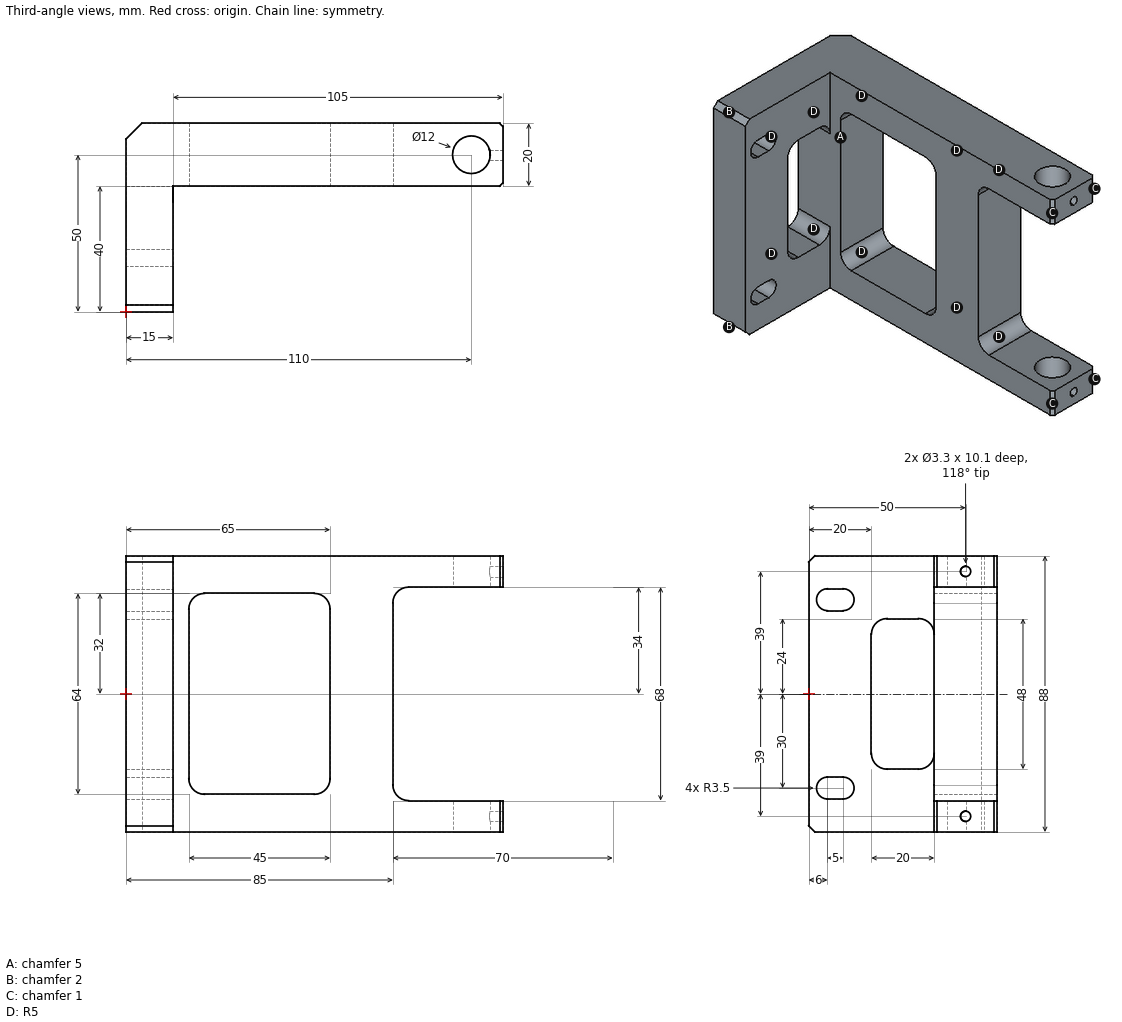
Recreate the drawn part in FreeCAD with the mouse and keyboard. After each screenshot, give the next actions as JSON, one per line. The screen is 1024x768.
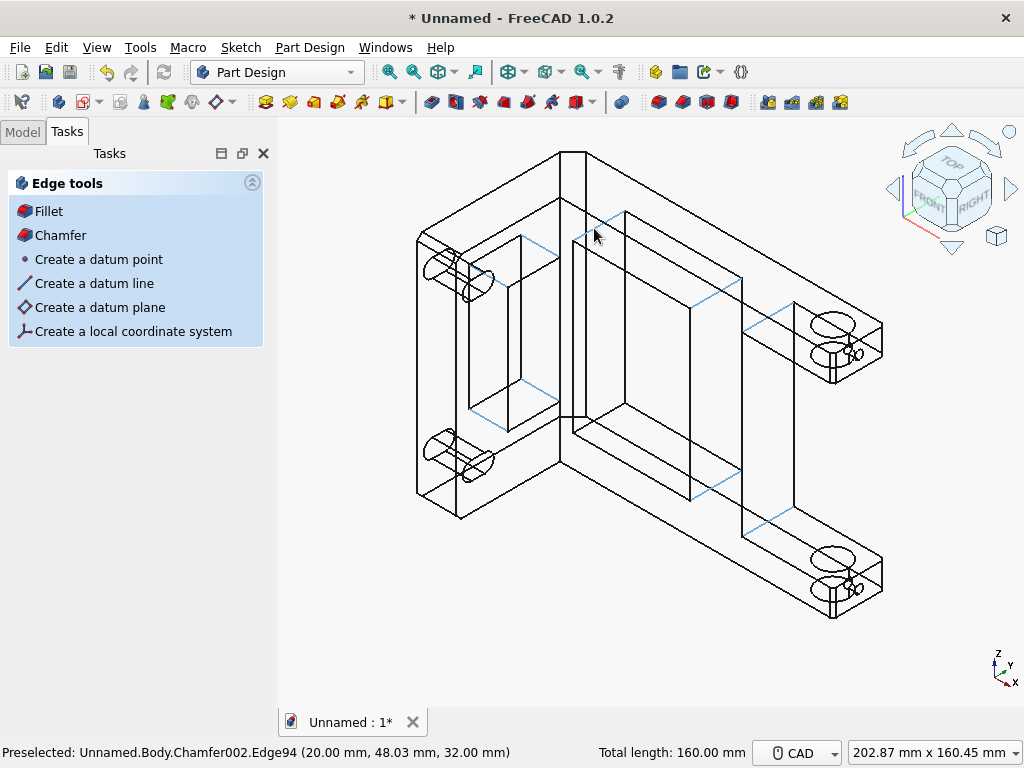
{"action": "left_click", "coordinate": [599, 417], "text": "ctrl"}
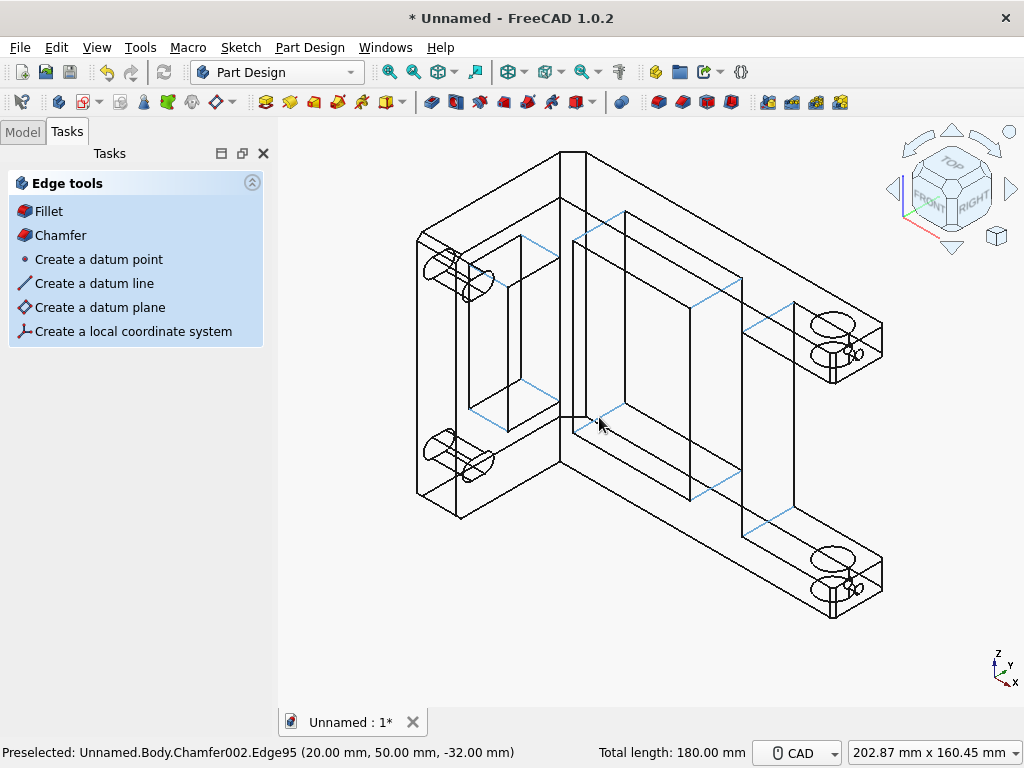
{"action": "key", "text": "v 1"}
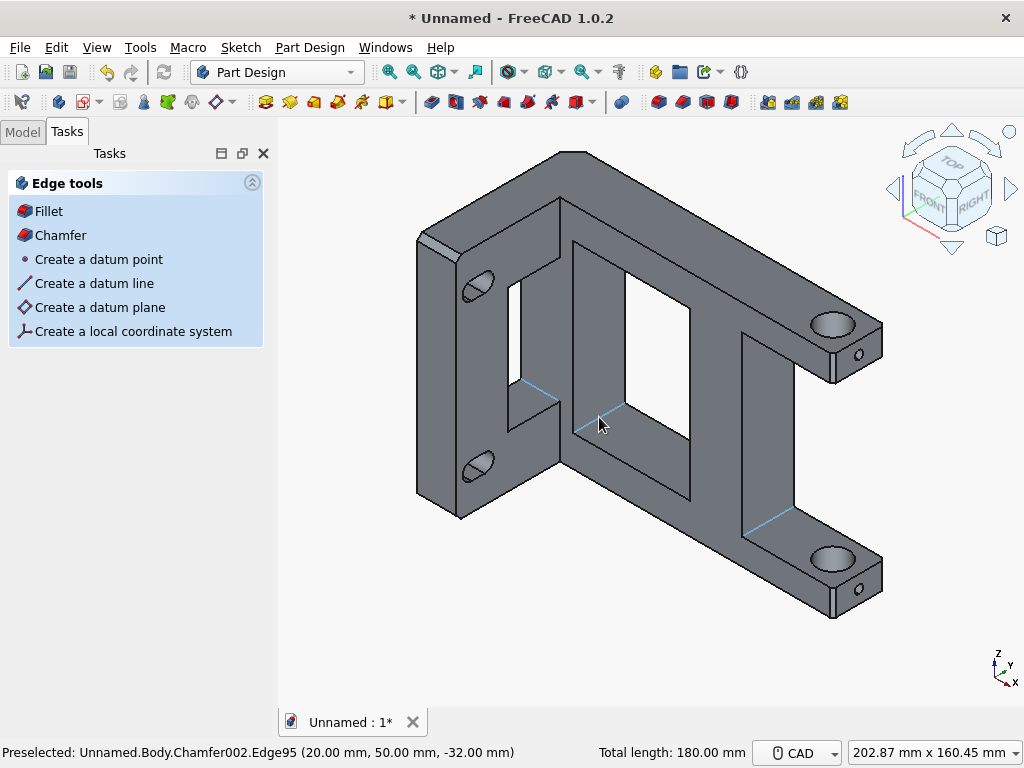
{"action": "left_click", "coordinate": [660, 102]}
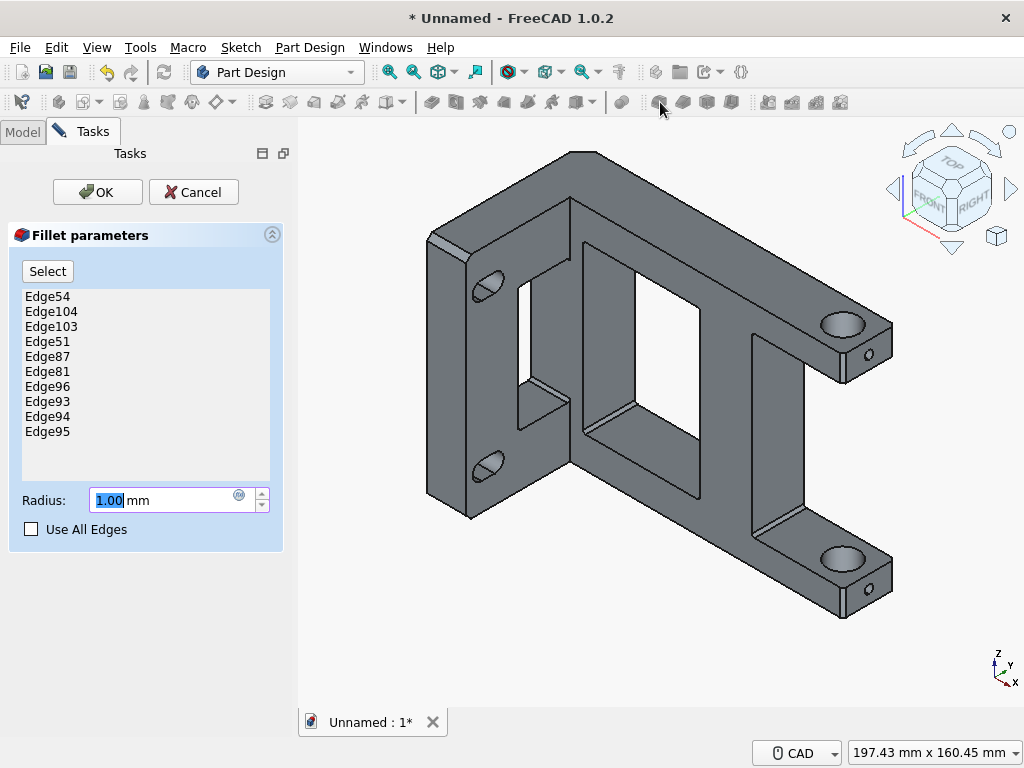
{"action": "type", "text": "5"}
{"action": "key", "text": "Tab"}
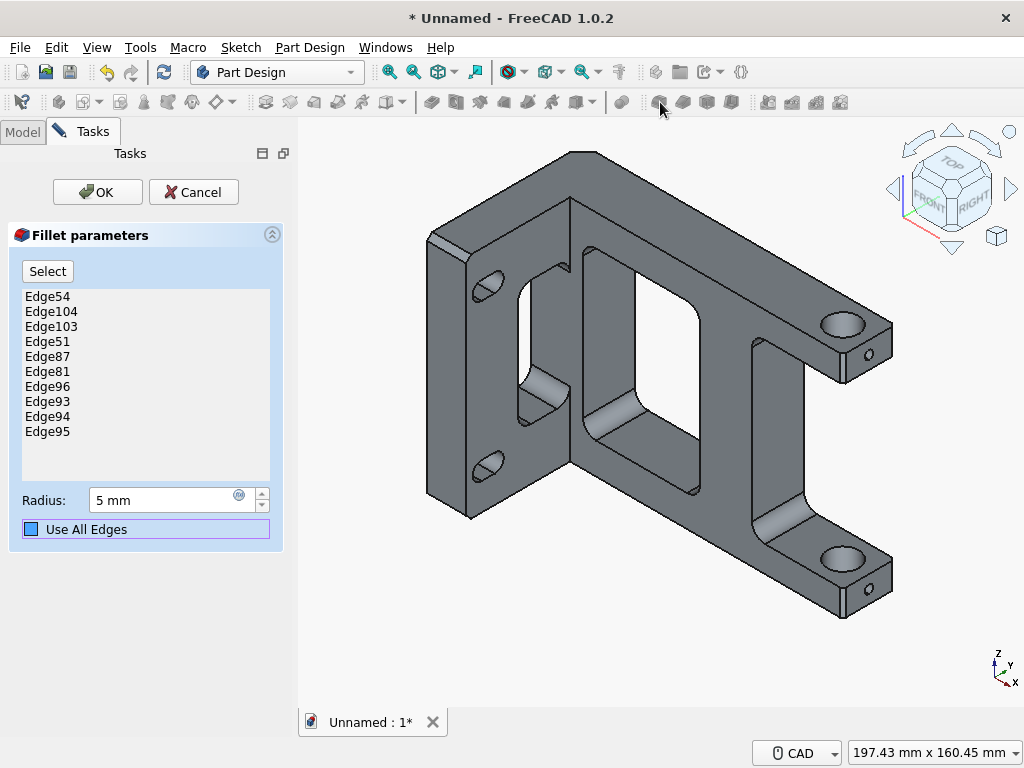
{"action": "left_click", "coordinate": [98, 192]}